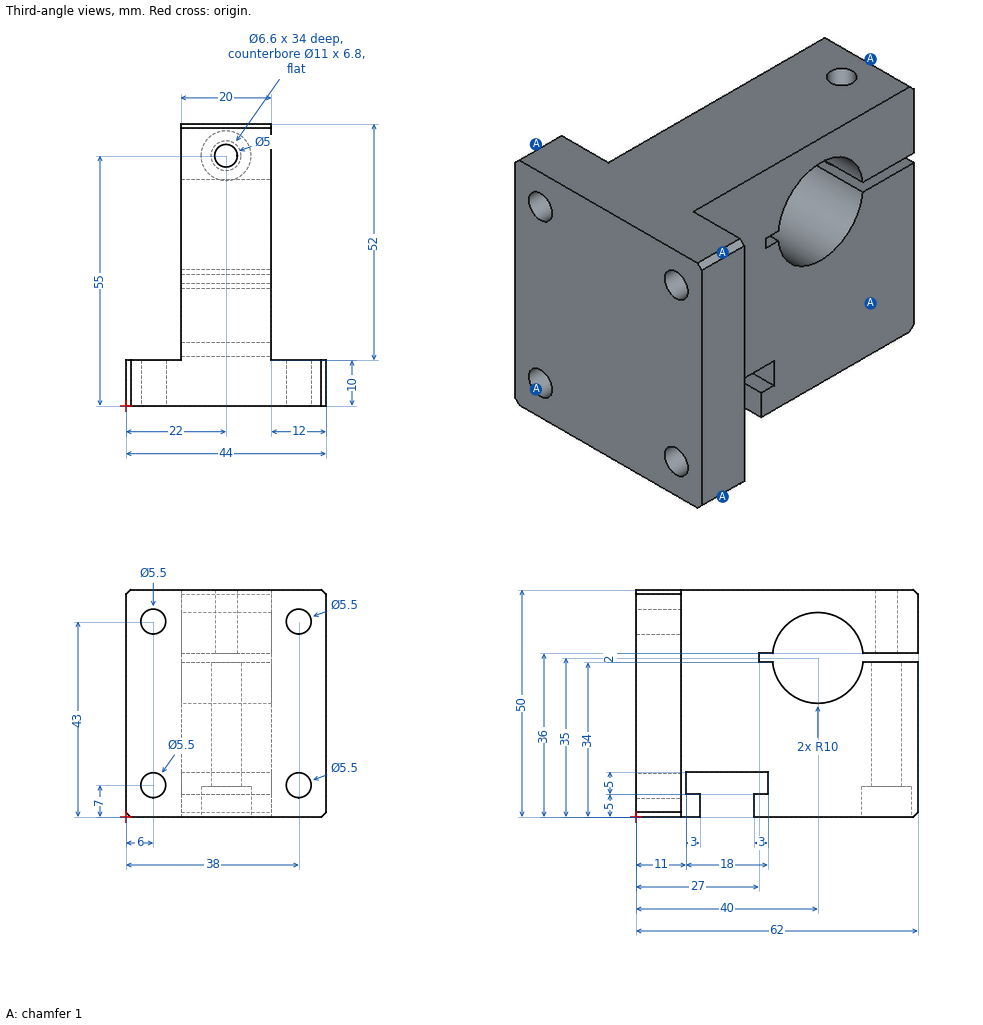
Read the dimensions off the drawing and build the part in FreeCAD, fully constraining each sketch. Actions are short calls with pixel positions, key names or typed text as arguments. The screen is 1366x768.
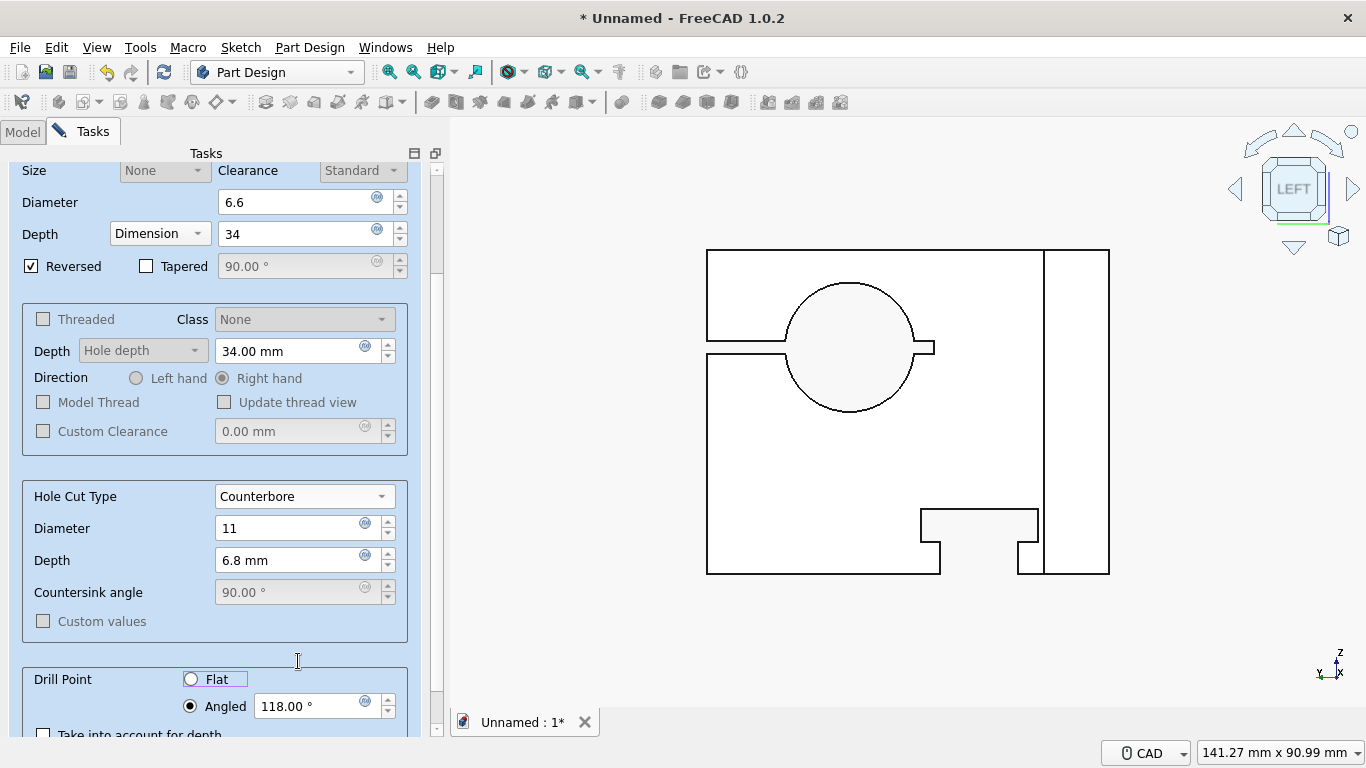
click(191, 679)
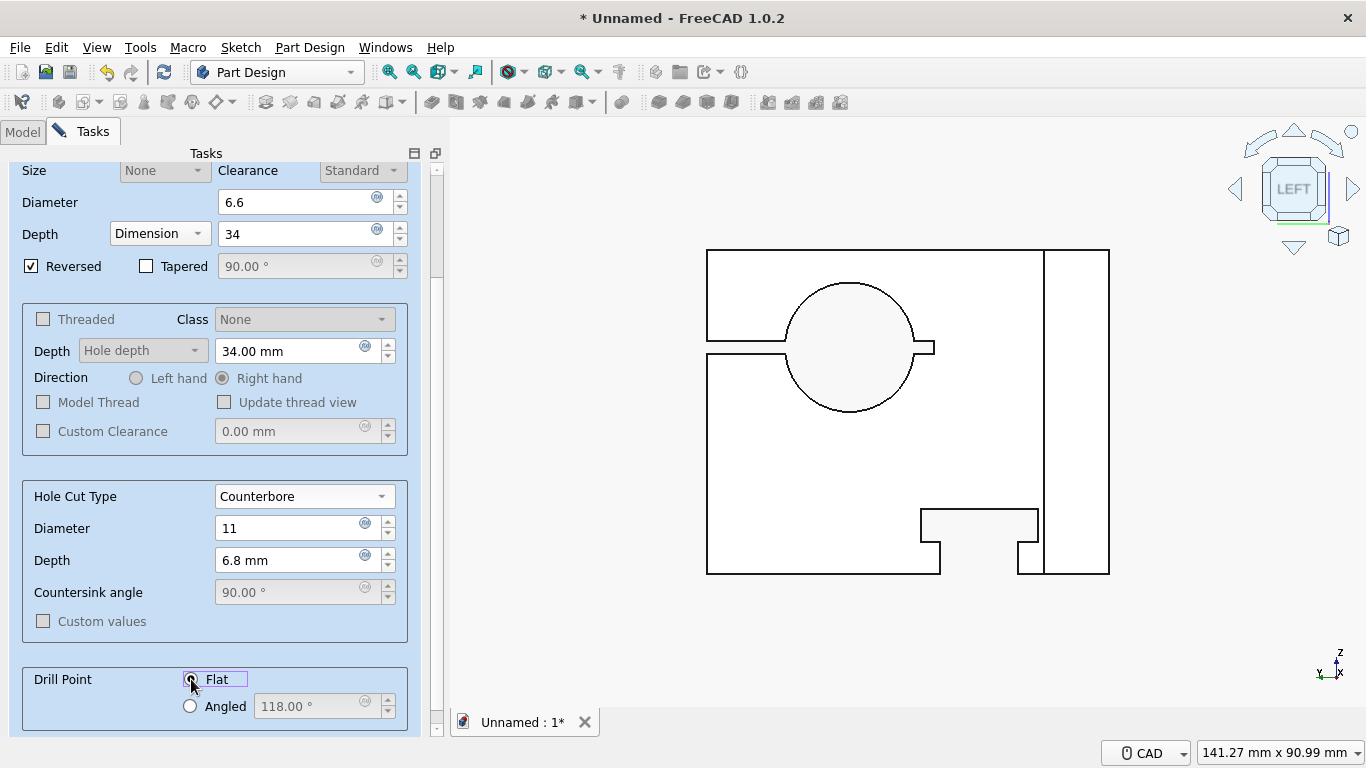
scroll(437, 450, up, 3)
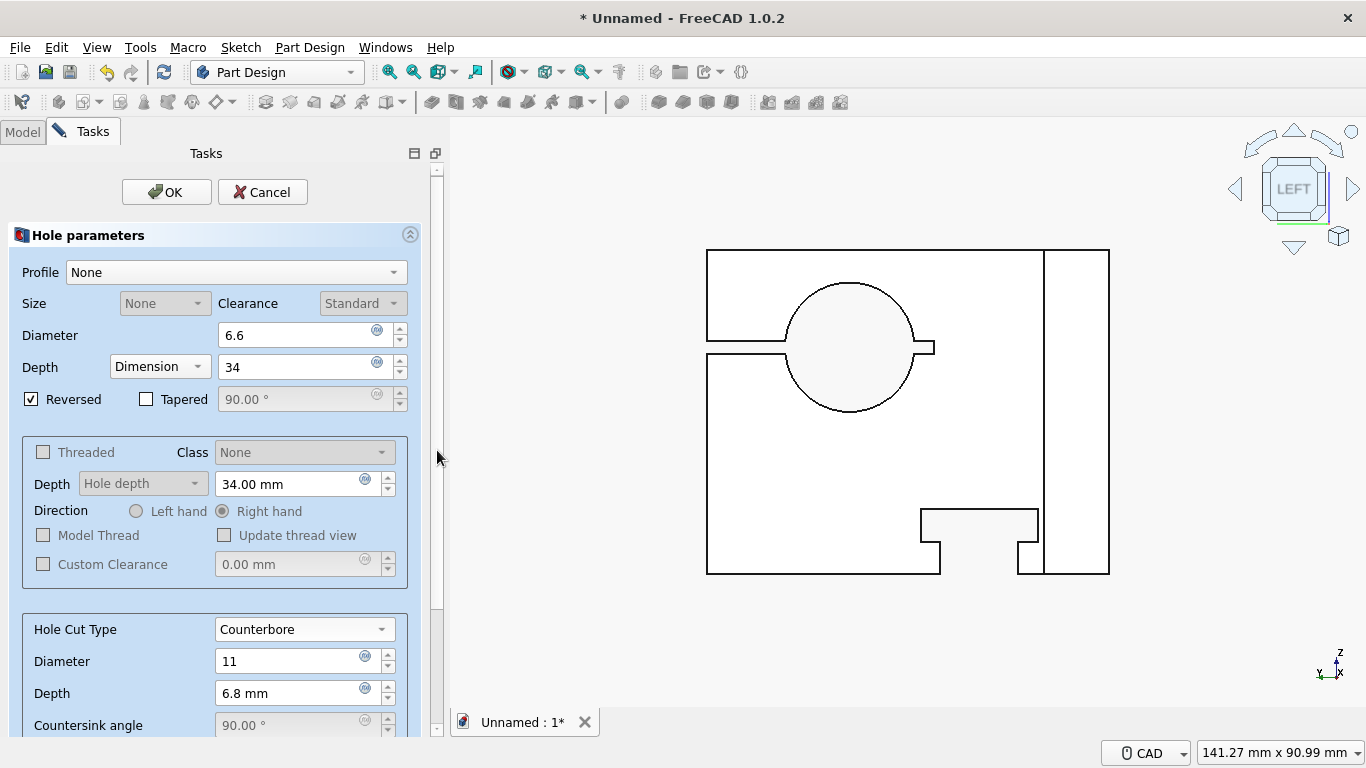
click(167, 192)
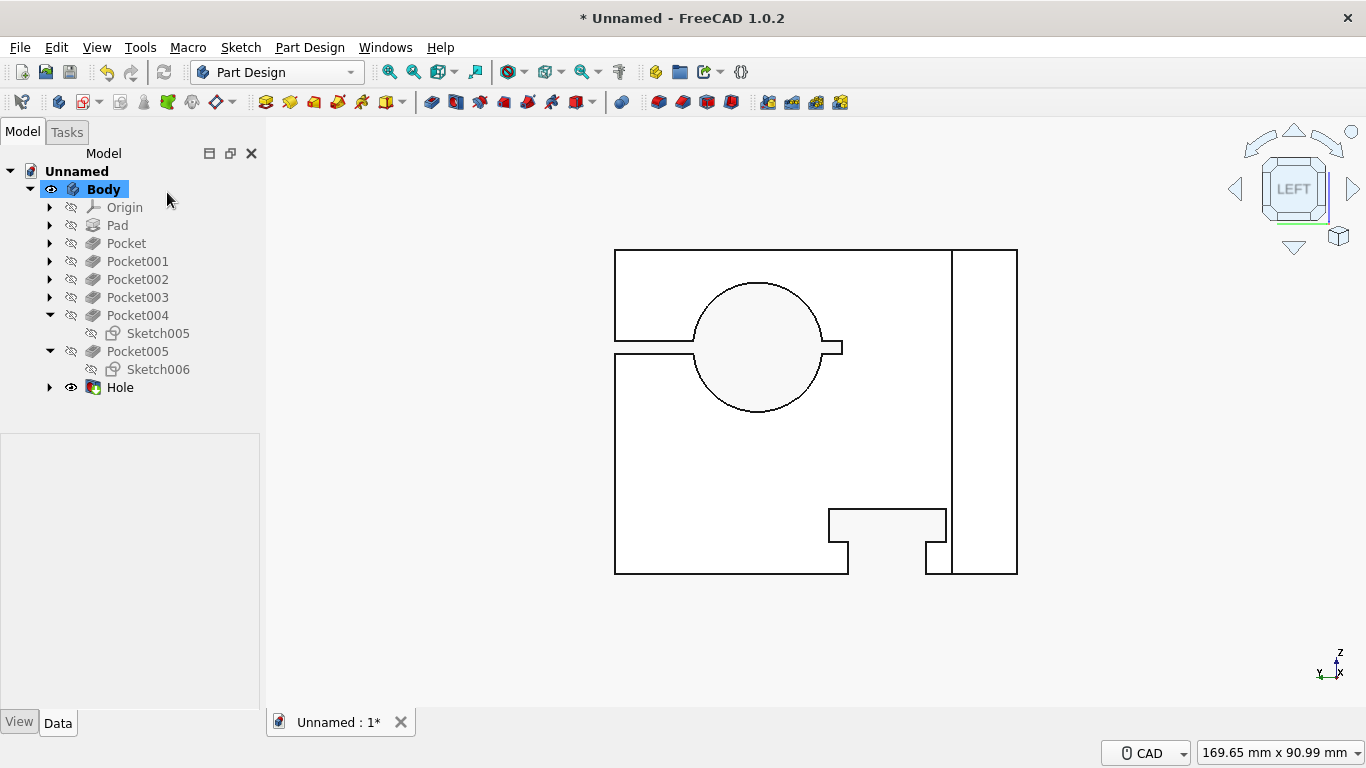
key(5)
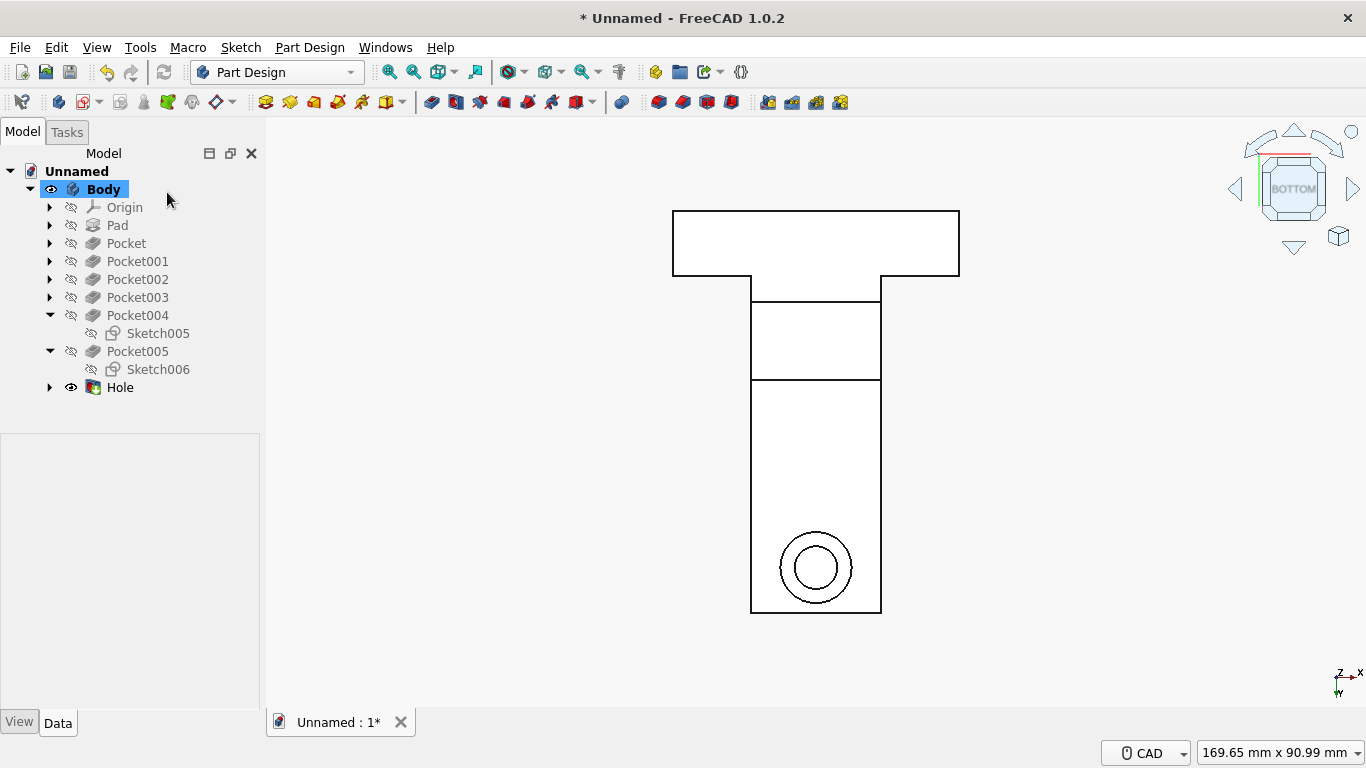
click(816, 462)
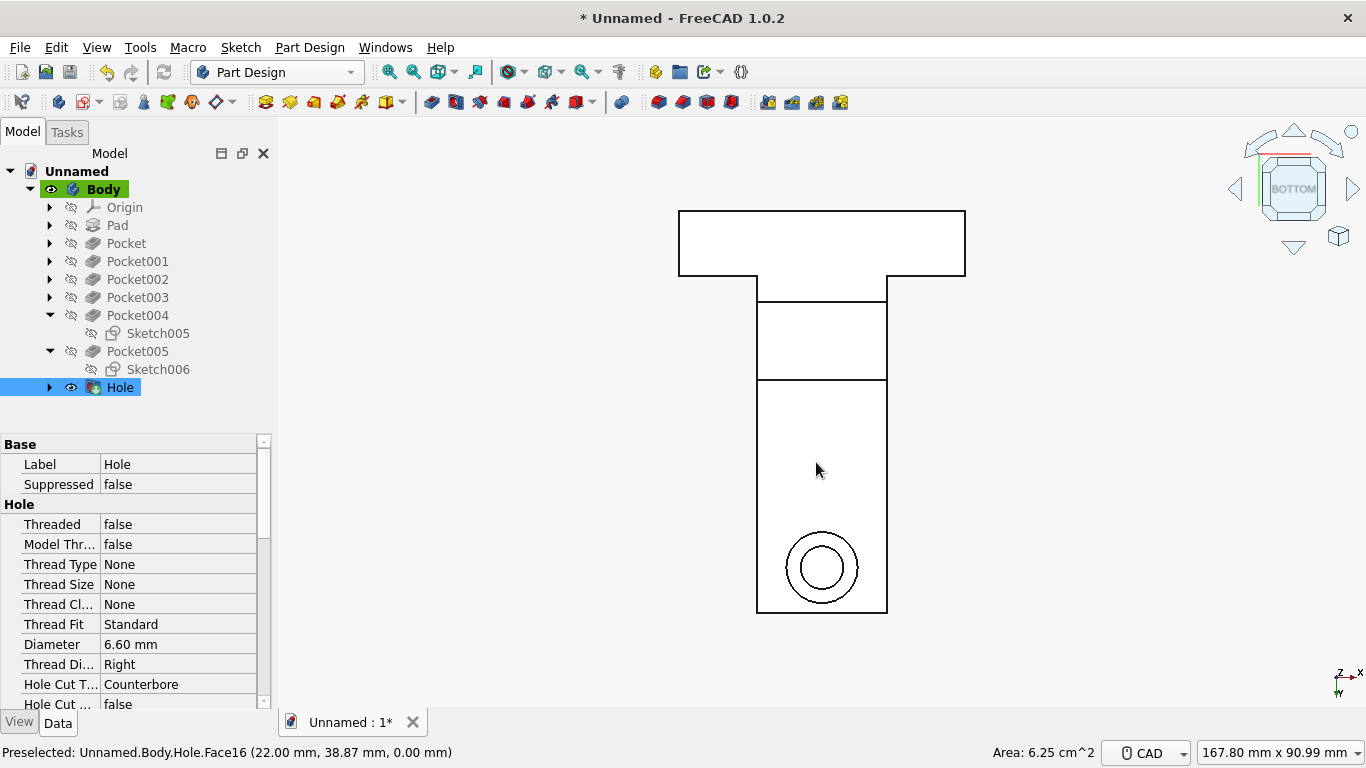
click(84, 102)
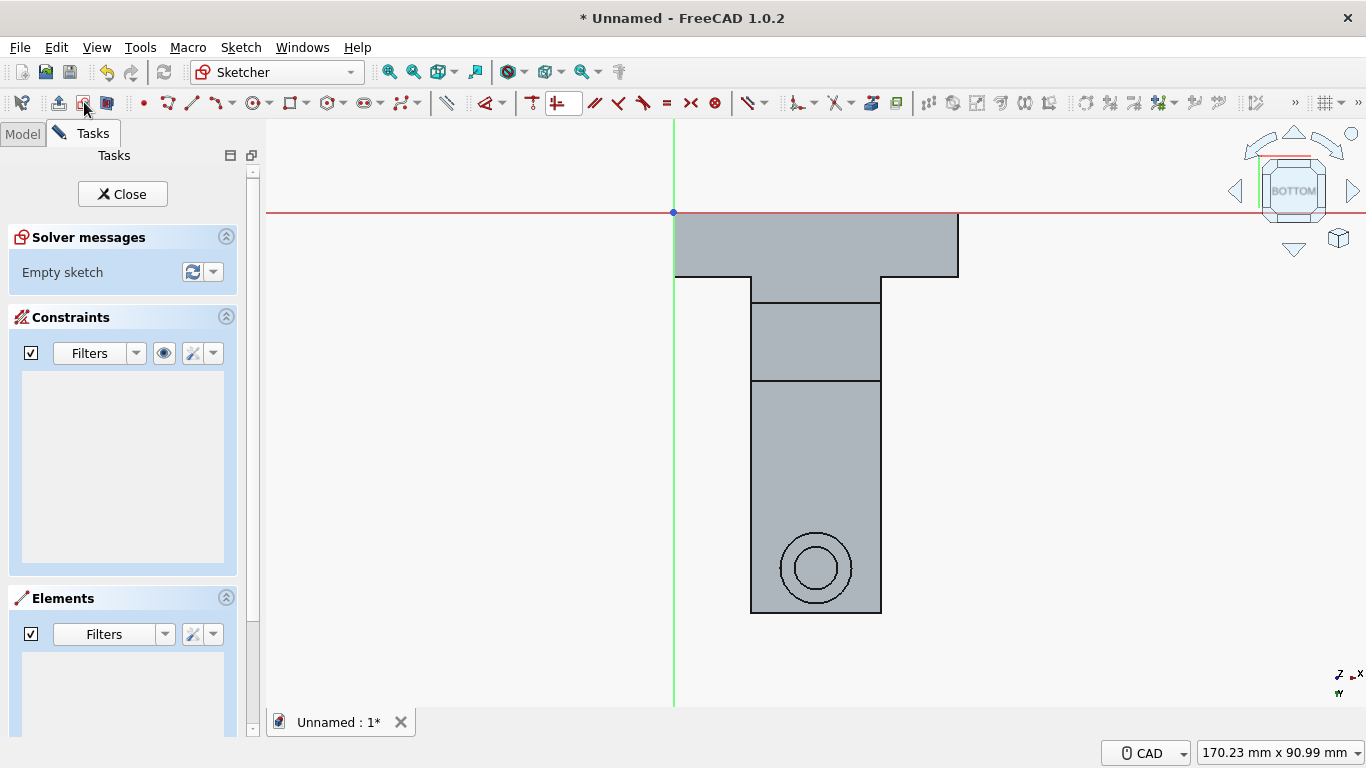
scroll(823, 584, up, 12)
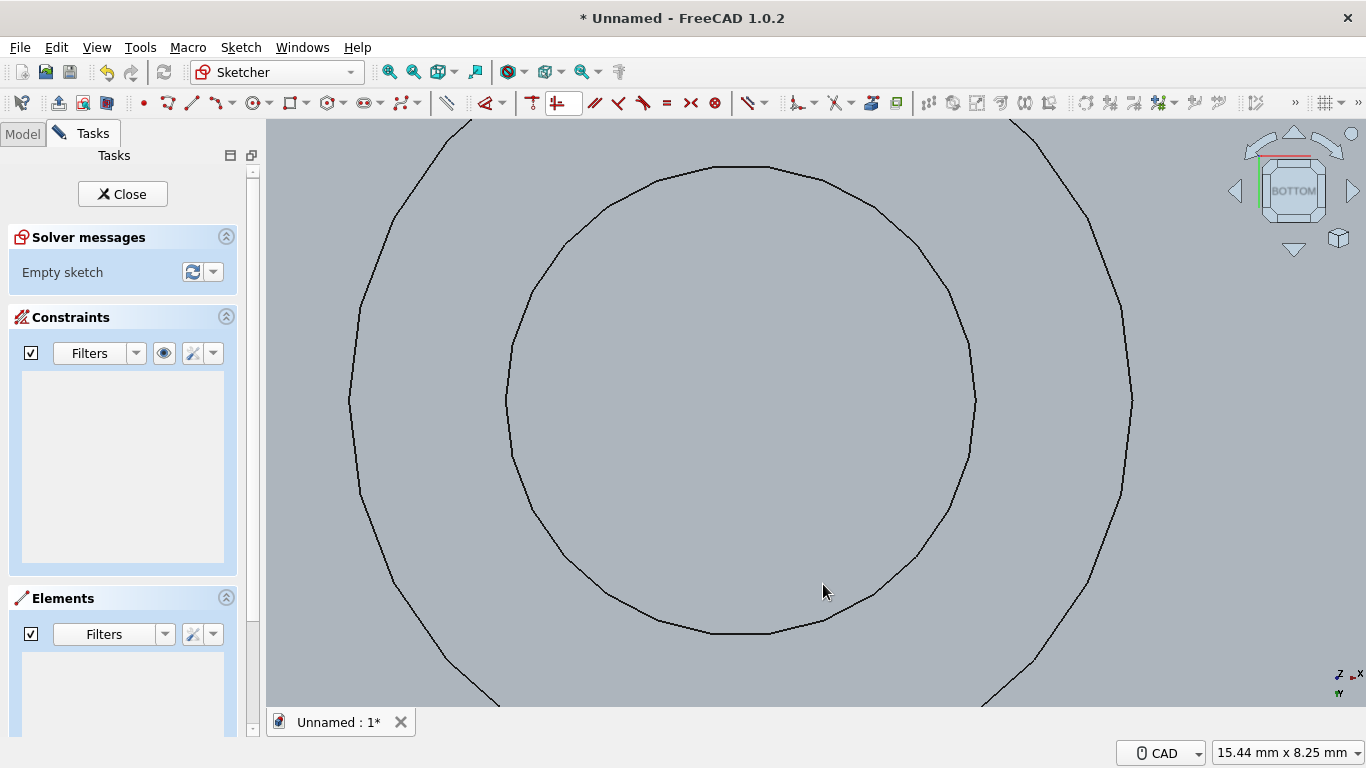
click(254, 104)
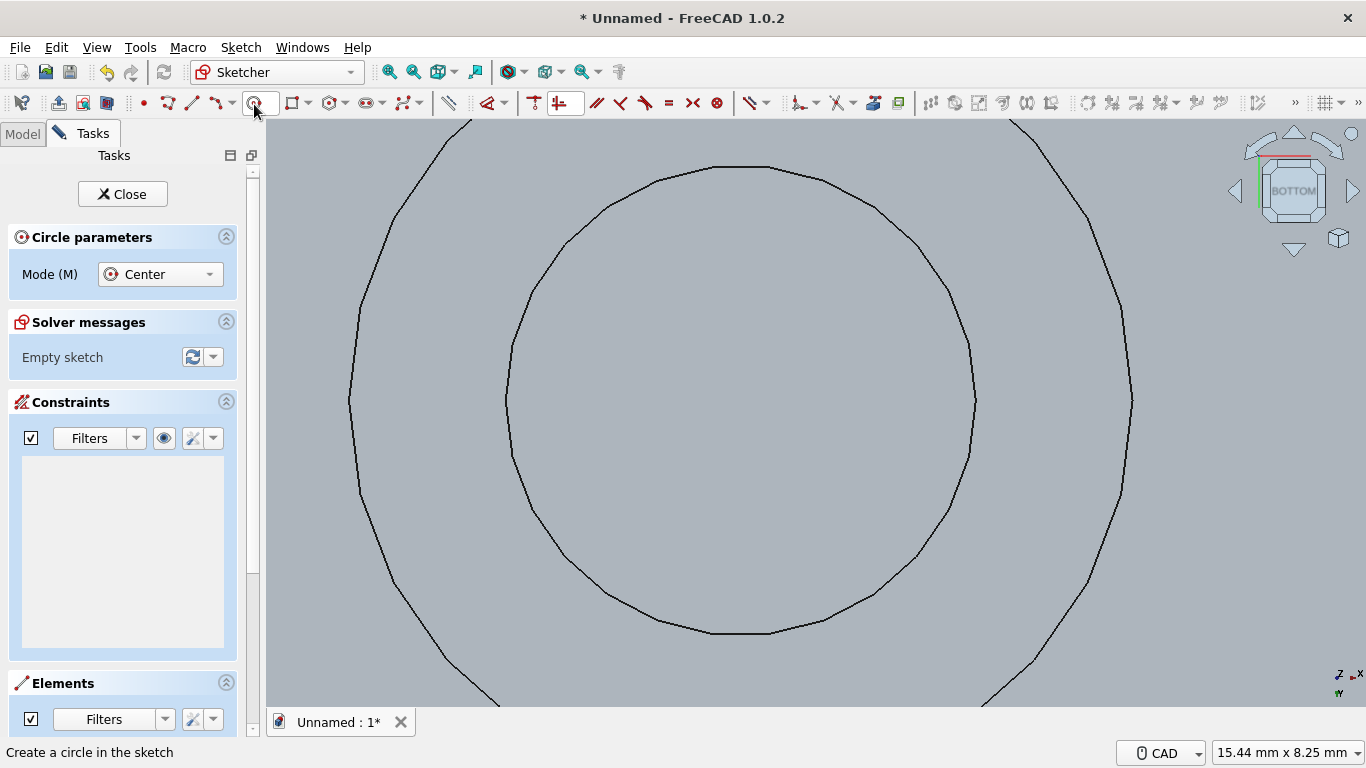
click(741, 401)
move(867, 275)